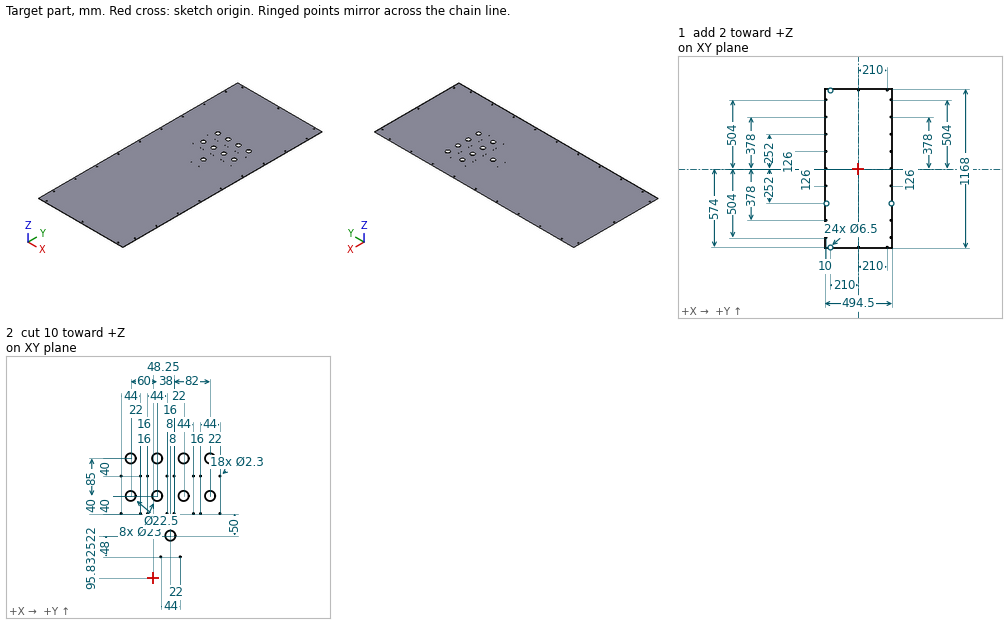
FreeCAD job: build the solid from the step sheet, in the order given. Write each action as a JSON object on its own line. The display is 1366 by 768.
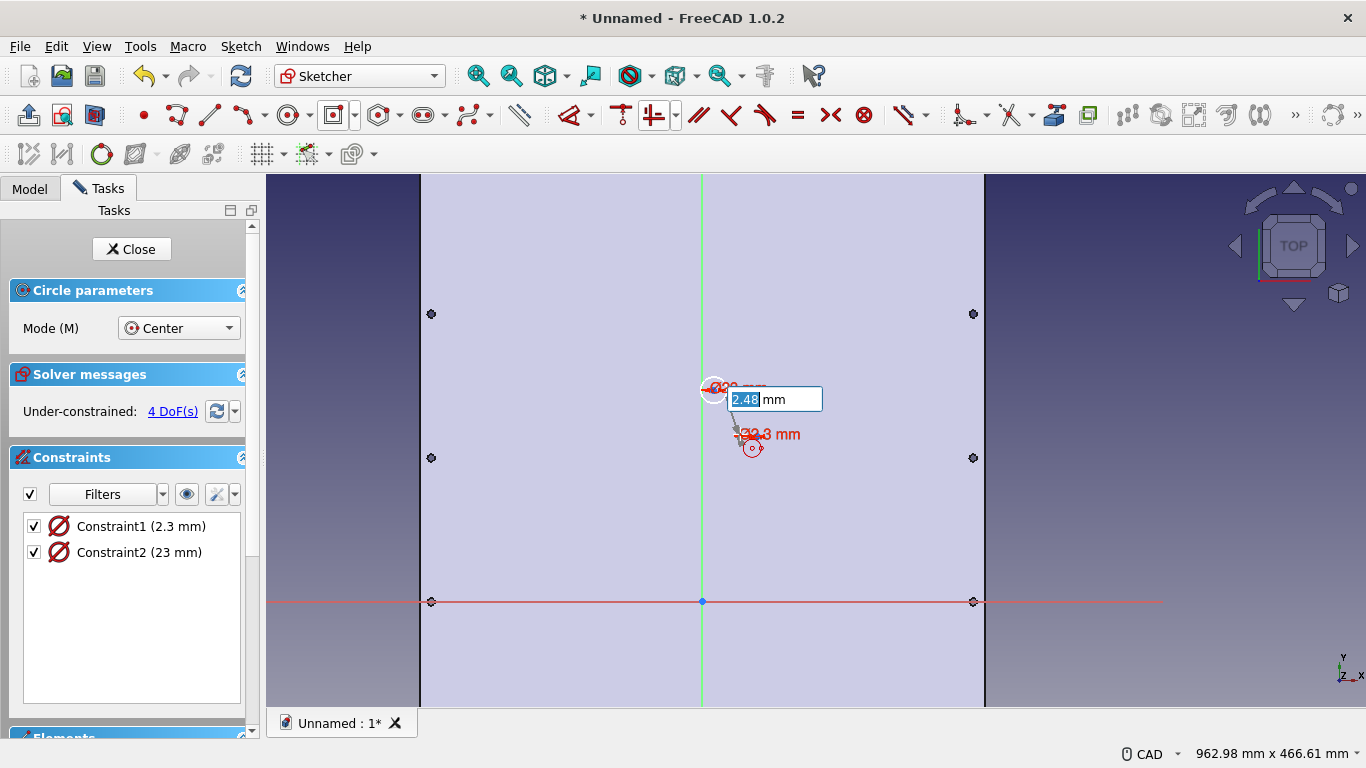
{"action": "type", "text": "2.3"}
{"action": "key", "text": "Return"}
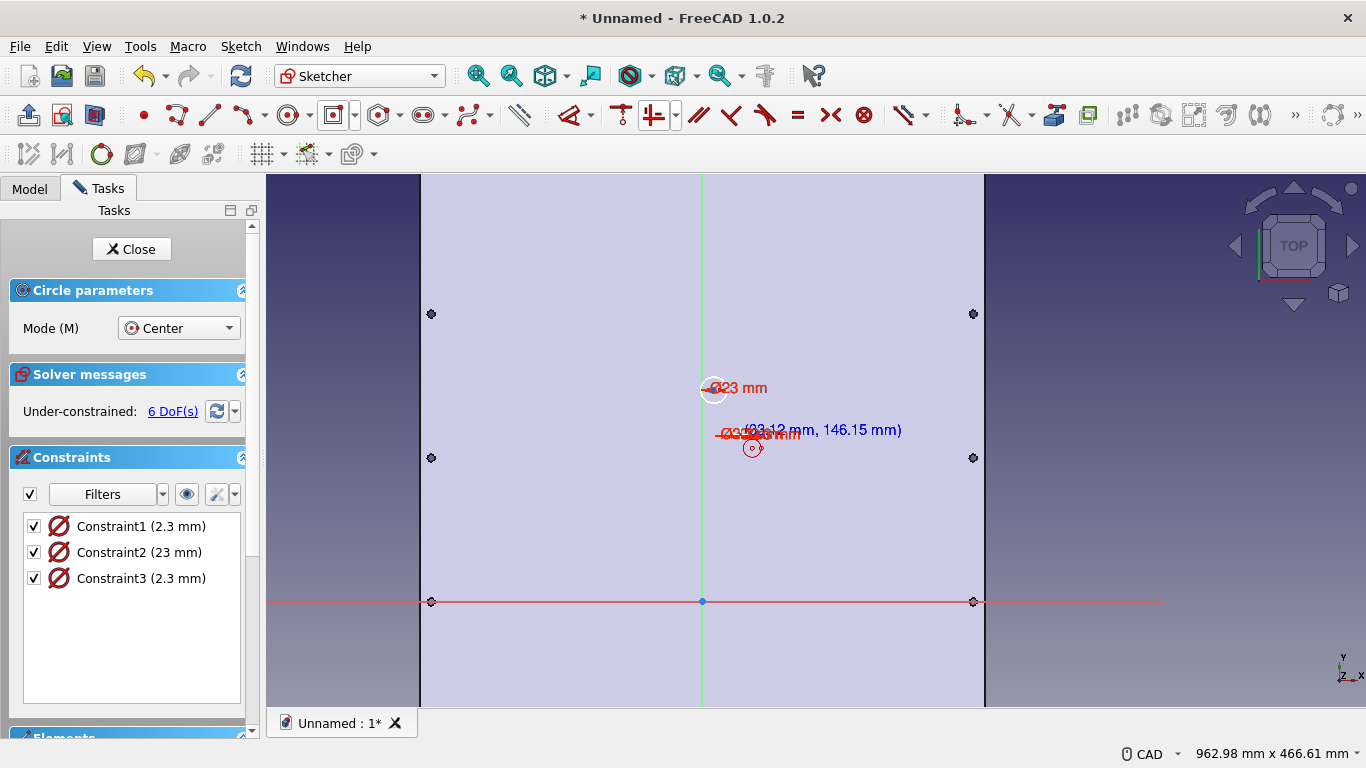
{"action": "scroll", "coordinate": [689, 435], "scroll_direction": "up", "scroll_amount": 15}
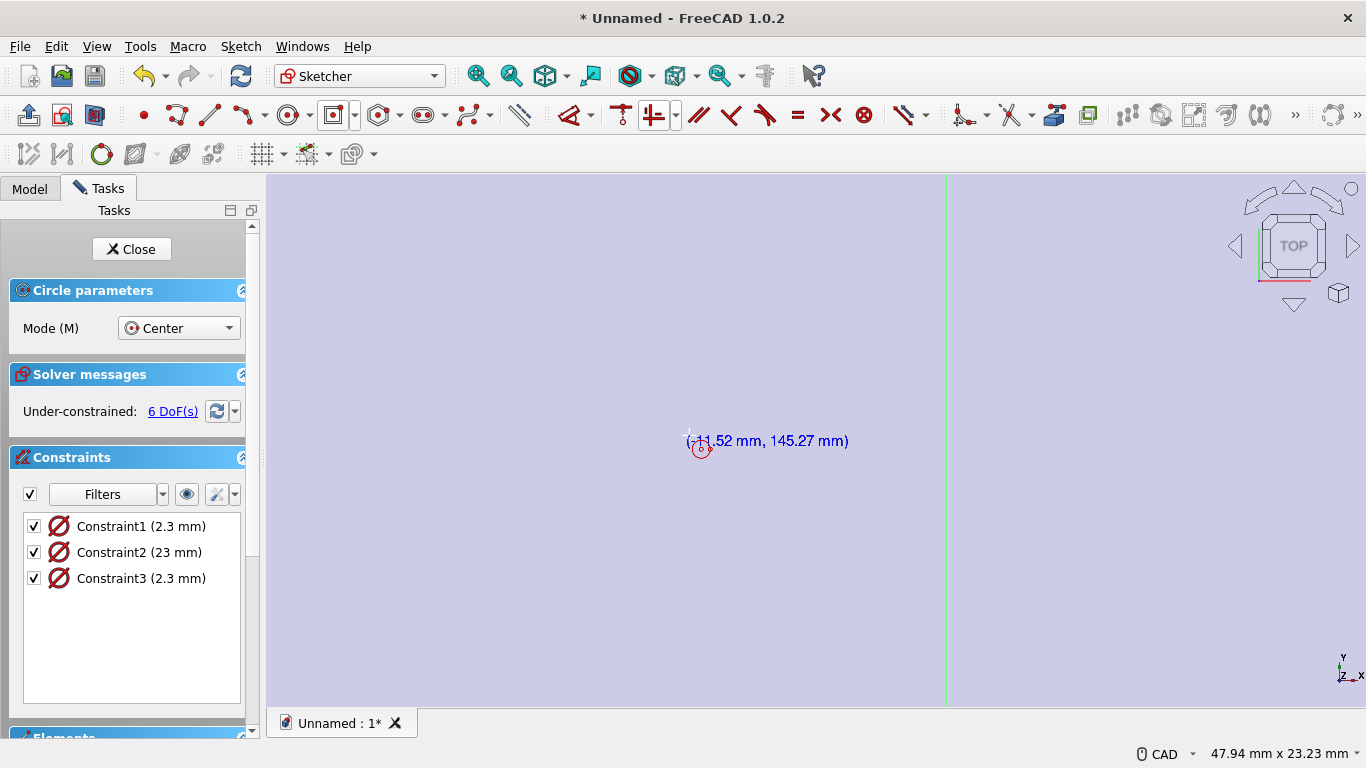
{"action": "scroll", "coordinate": [689, 435], "scroll_direction": "down", "scroll_amount": 15}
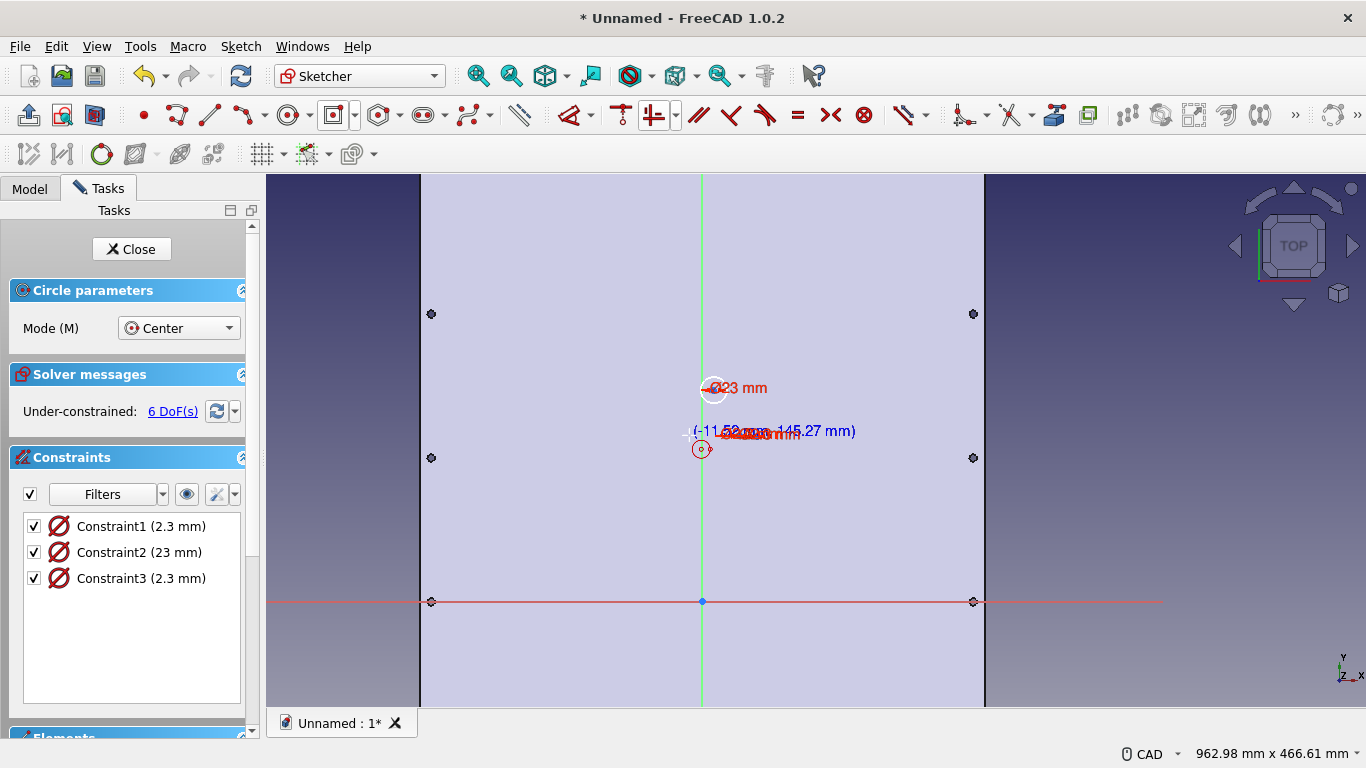
{"action": "left_click", "coordinate": [689, 435]}
{"action": "mouse_move", "coordinate": [688, 434]}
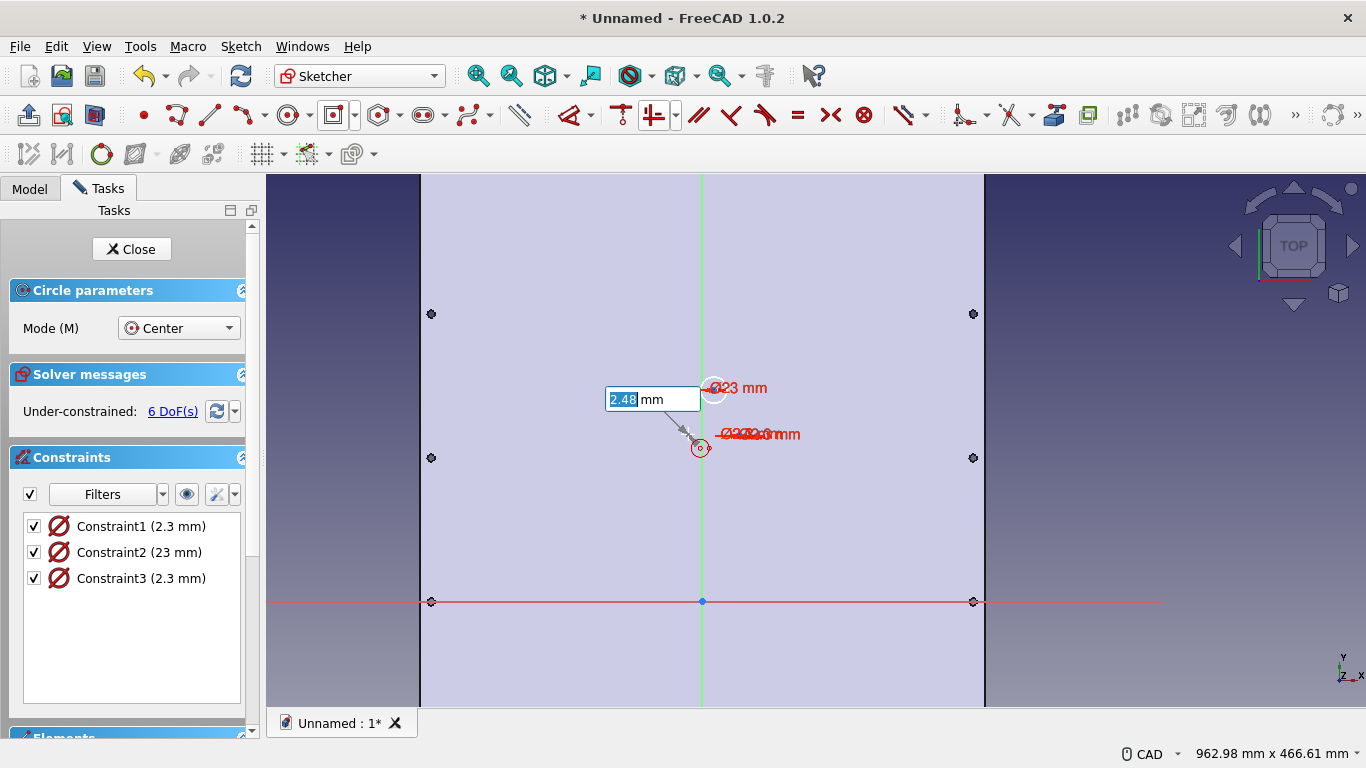
{"action": "type", "text": "2.3"}
{"action": "key", "text": "Return"}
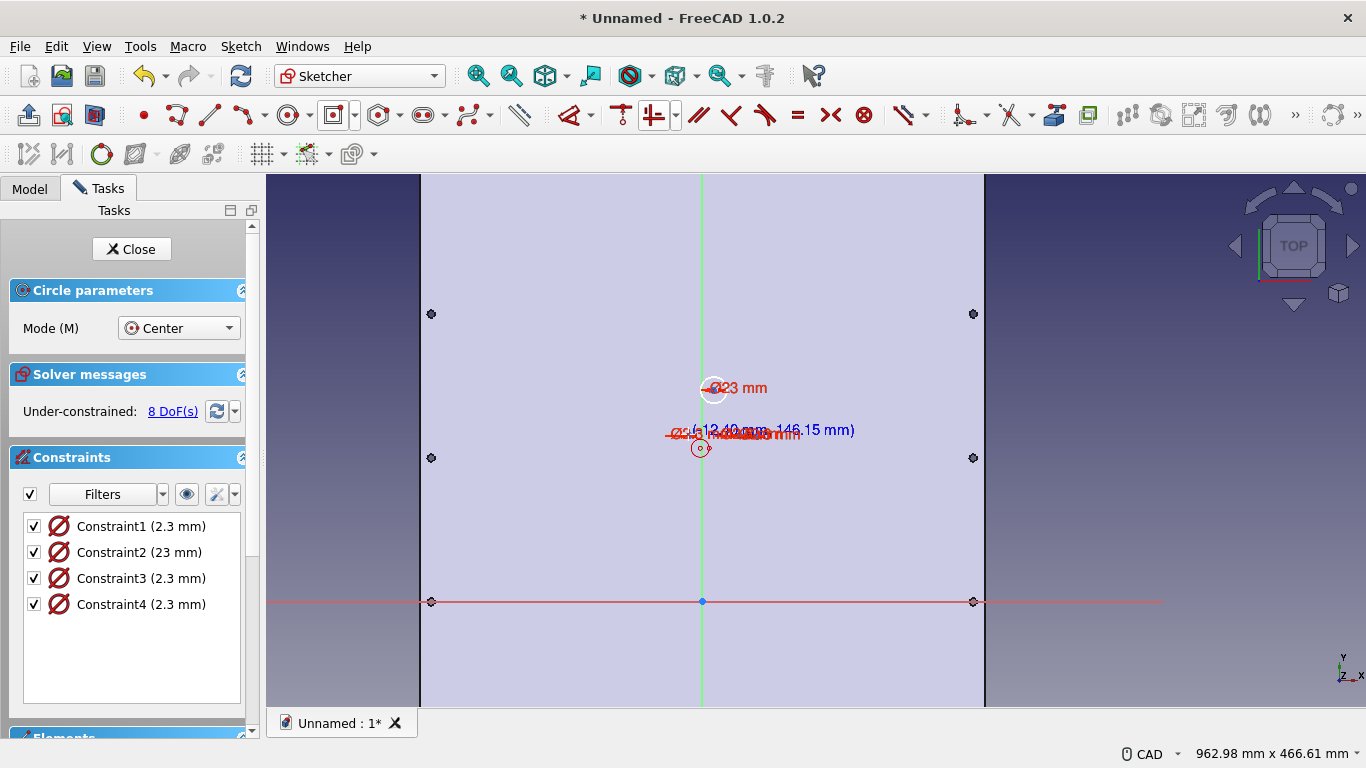
{"action": "scroll", "coordinate": [670, 435], "scroll_direction": "up", "scroll_amount": 15}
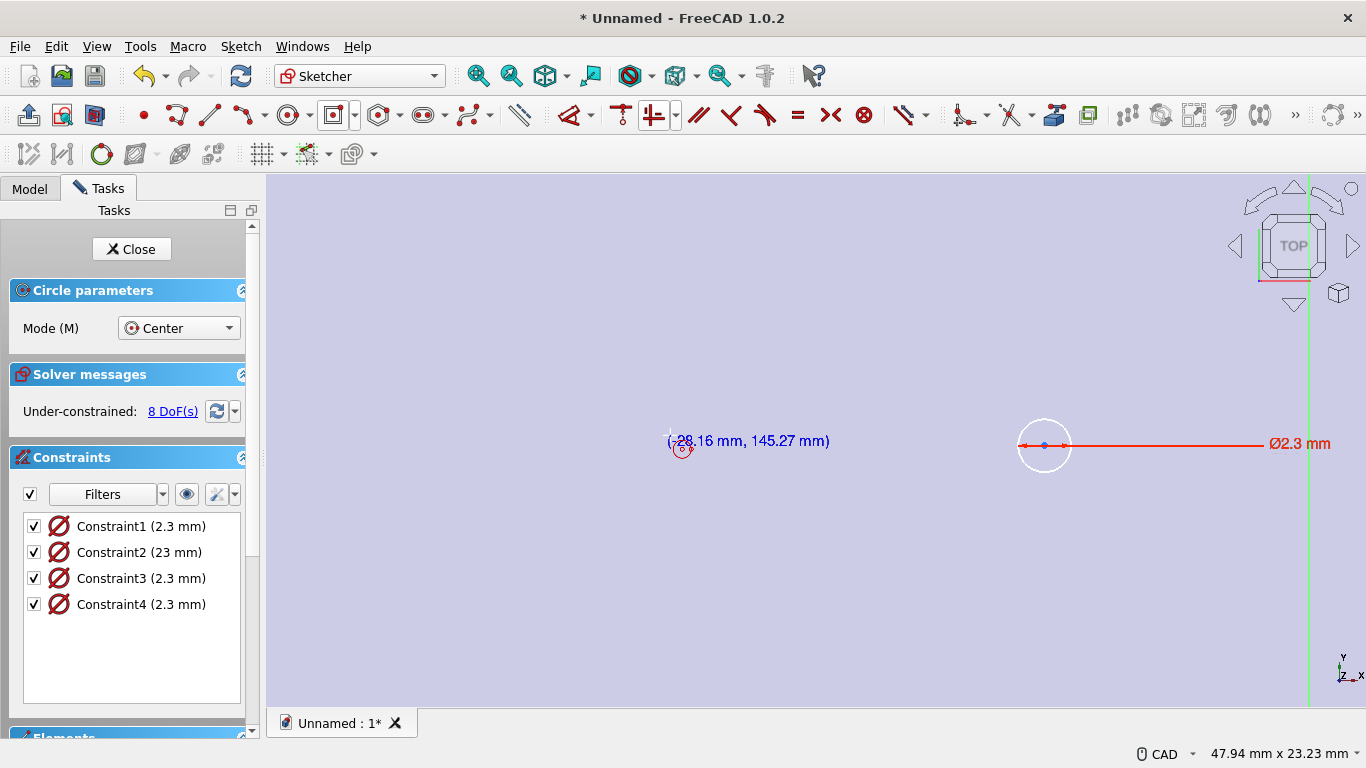
{"action": "scroll", "coordinate": [670, 435], "scroll_direction": "down", "scroll_amount": 15}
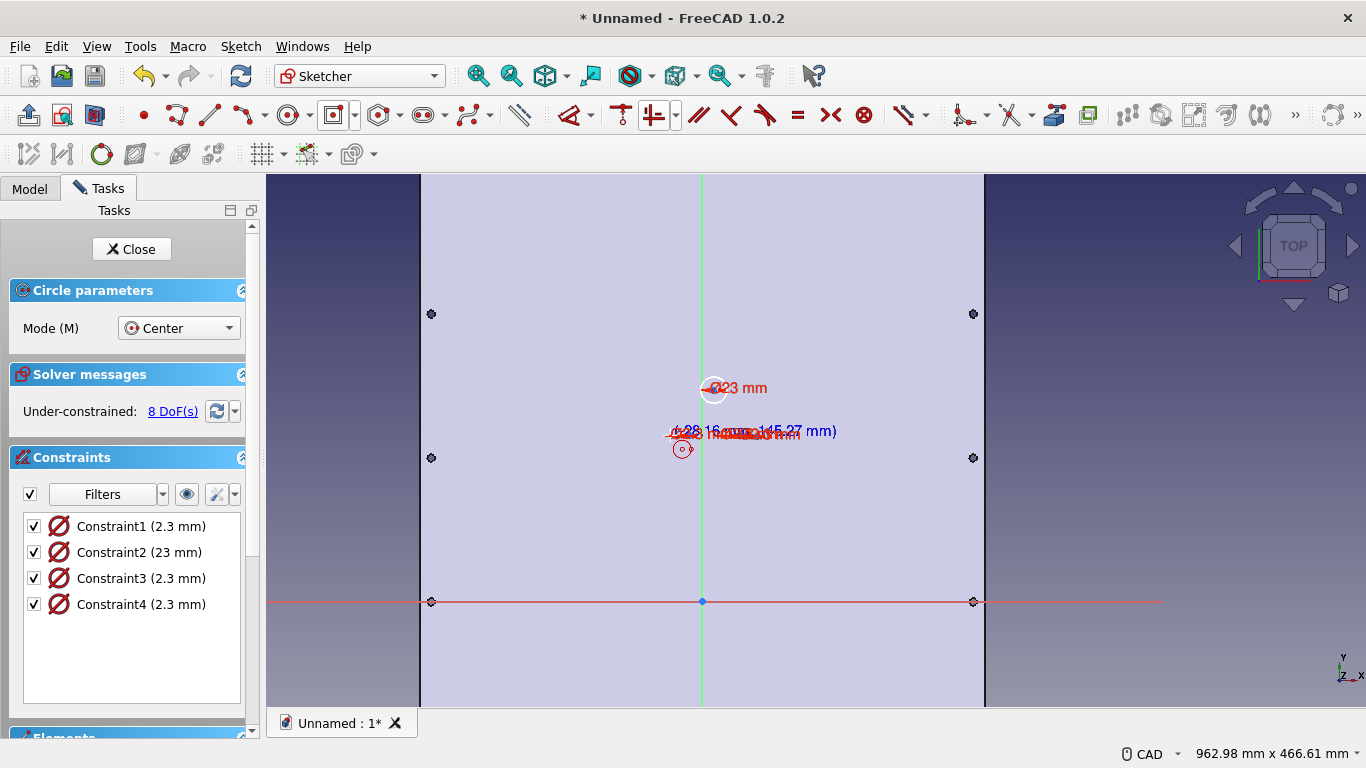
{"action": "left_click", "coordinate": [670, 435]}
{"action": "mouse_move", "coordinate": [671, 434]}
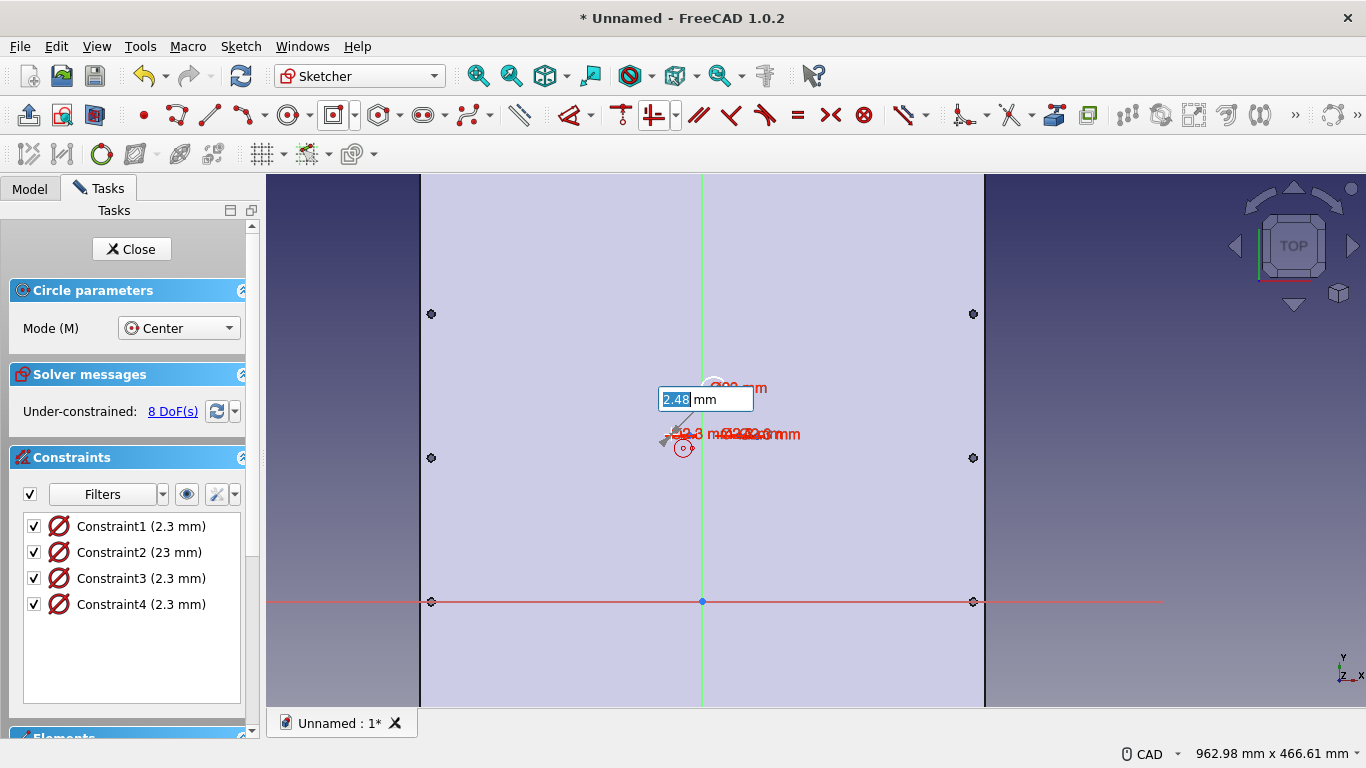
{"action": "type", "text": "2.3"}
{"action": "key", "text": "Return"}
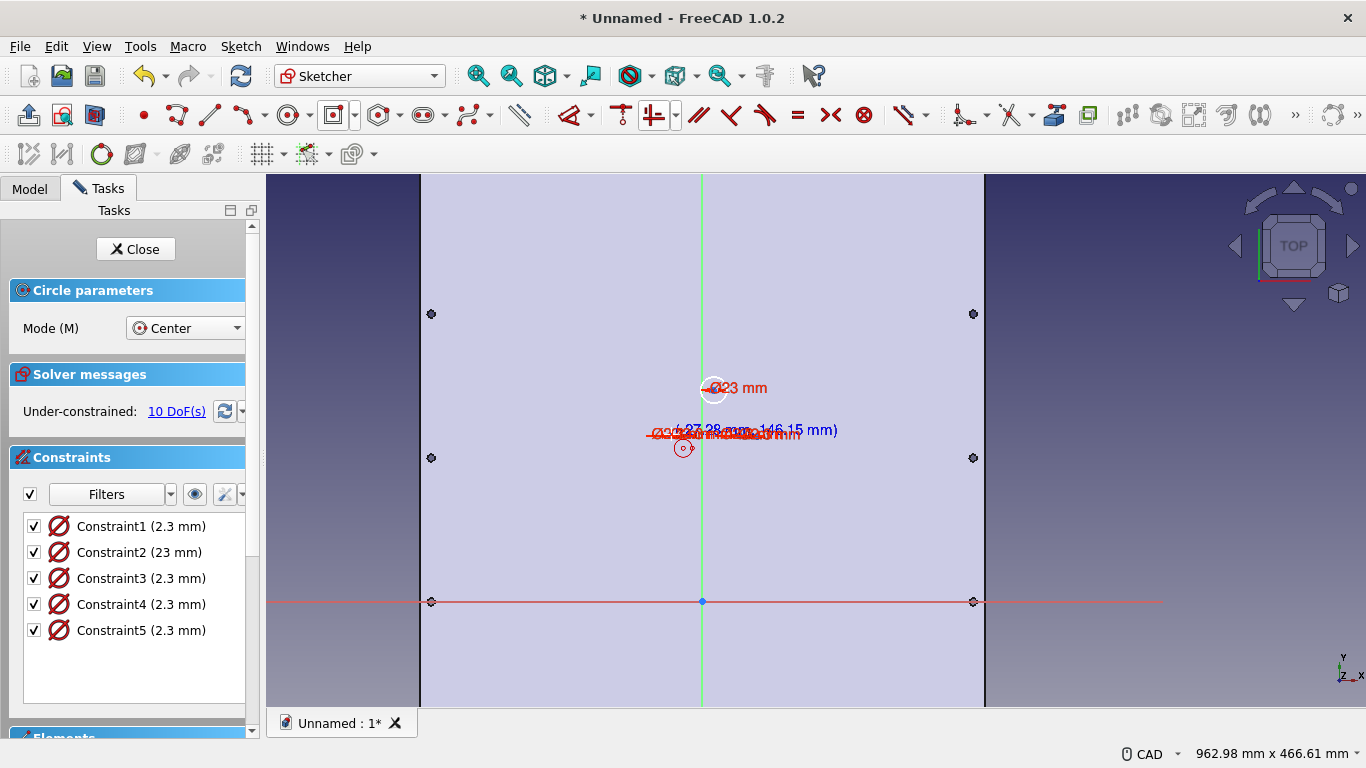
{"action": "scroll", "coordinate": [620, 435], "scroll_direction": "up", "scroll_amount": 15}